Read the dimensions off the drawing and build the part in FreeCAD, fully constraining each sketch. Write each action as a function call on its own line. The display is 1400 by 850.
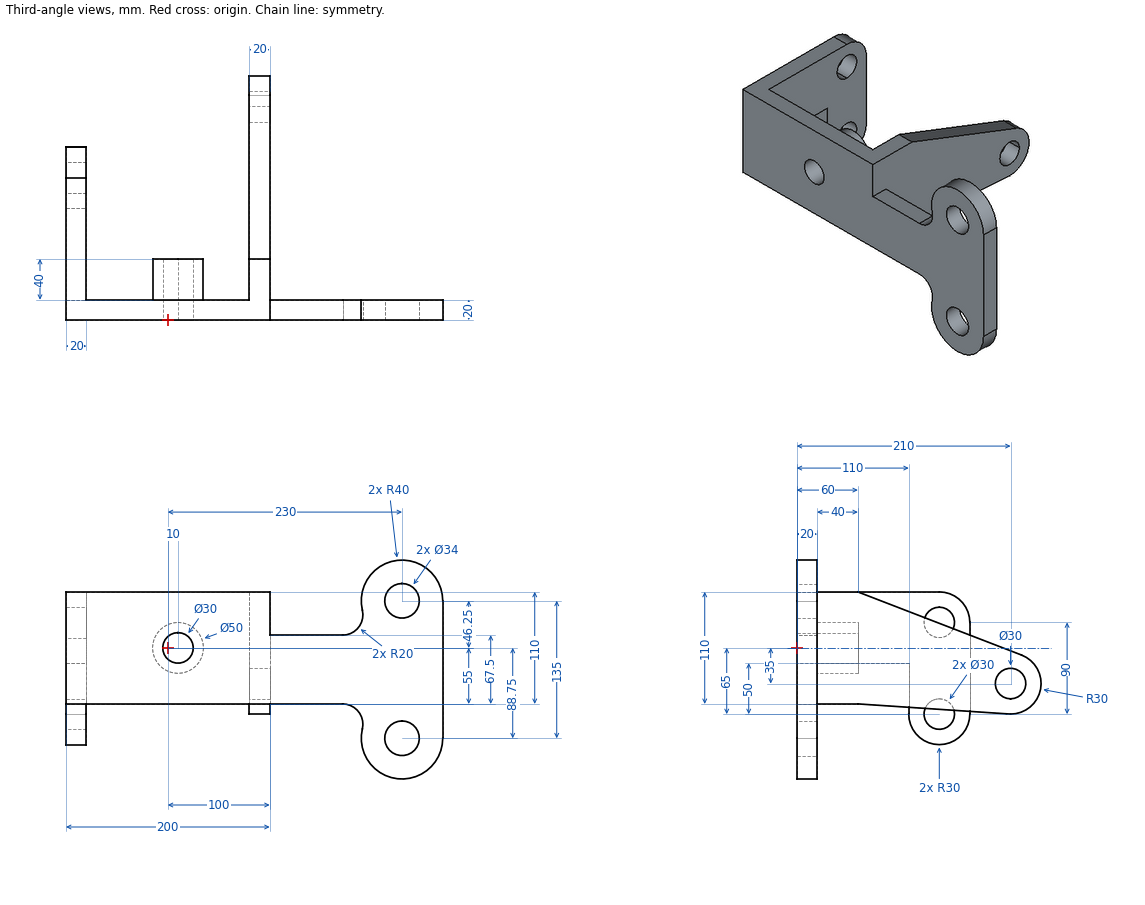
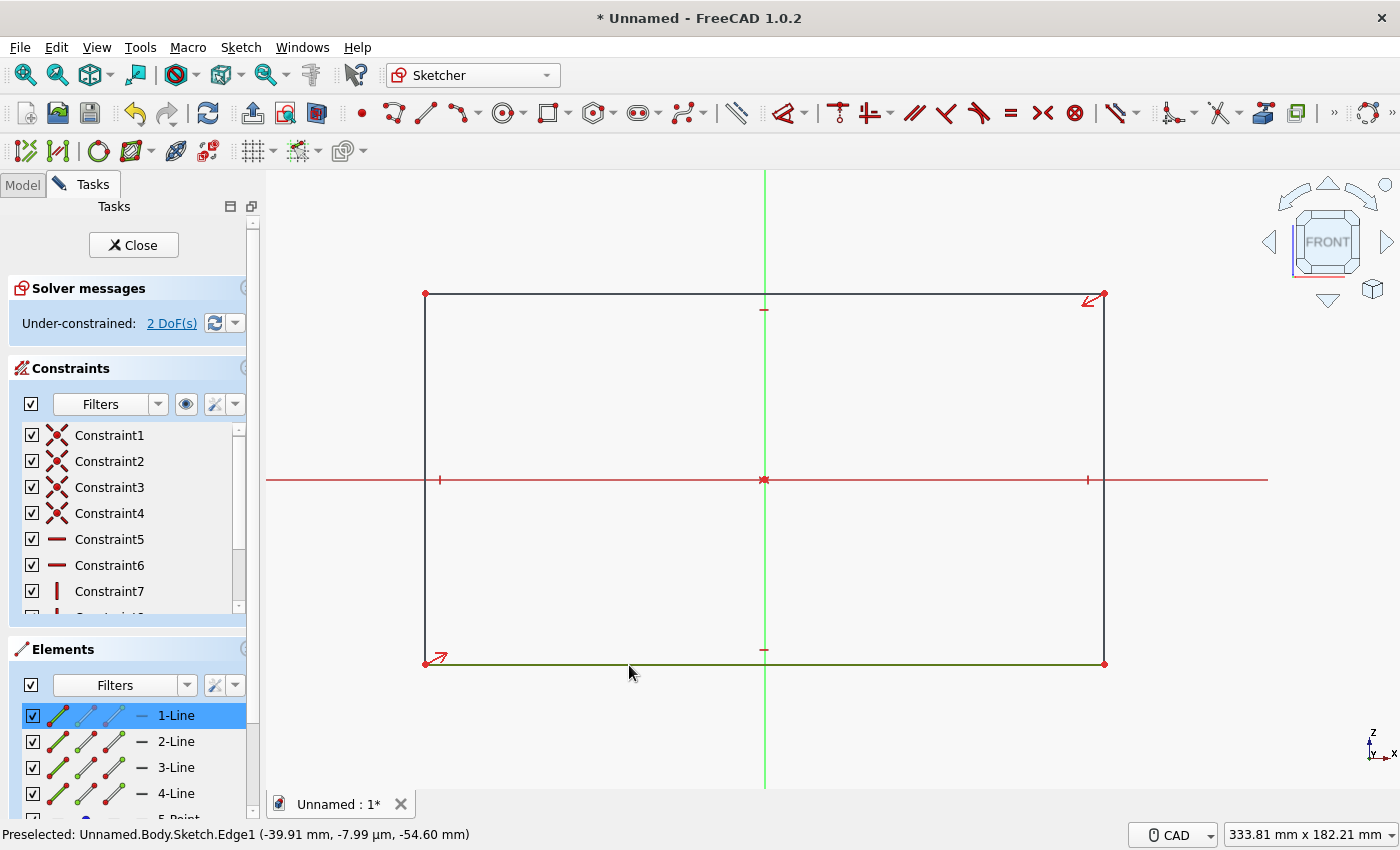
key(l)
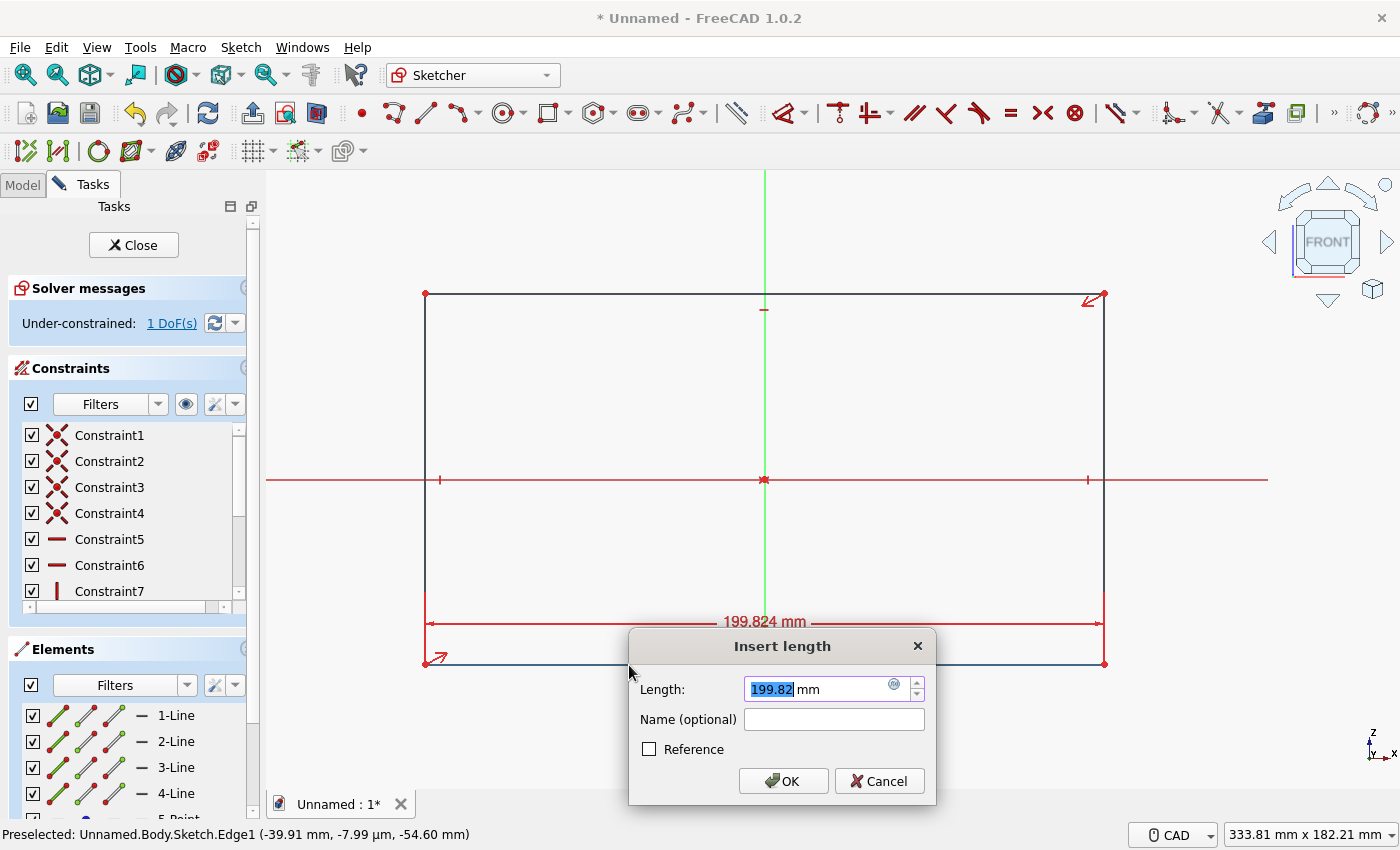
text(200)
key(Return)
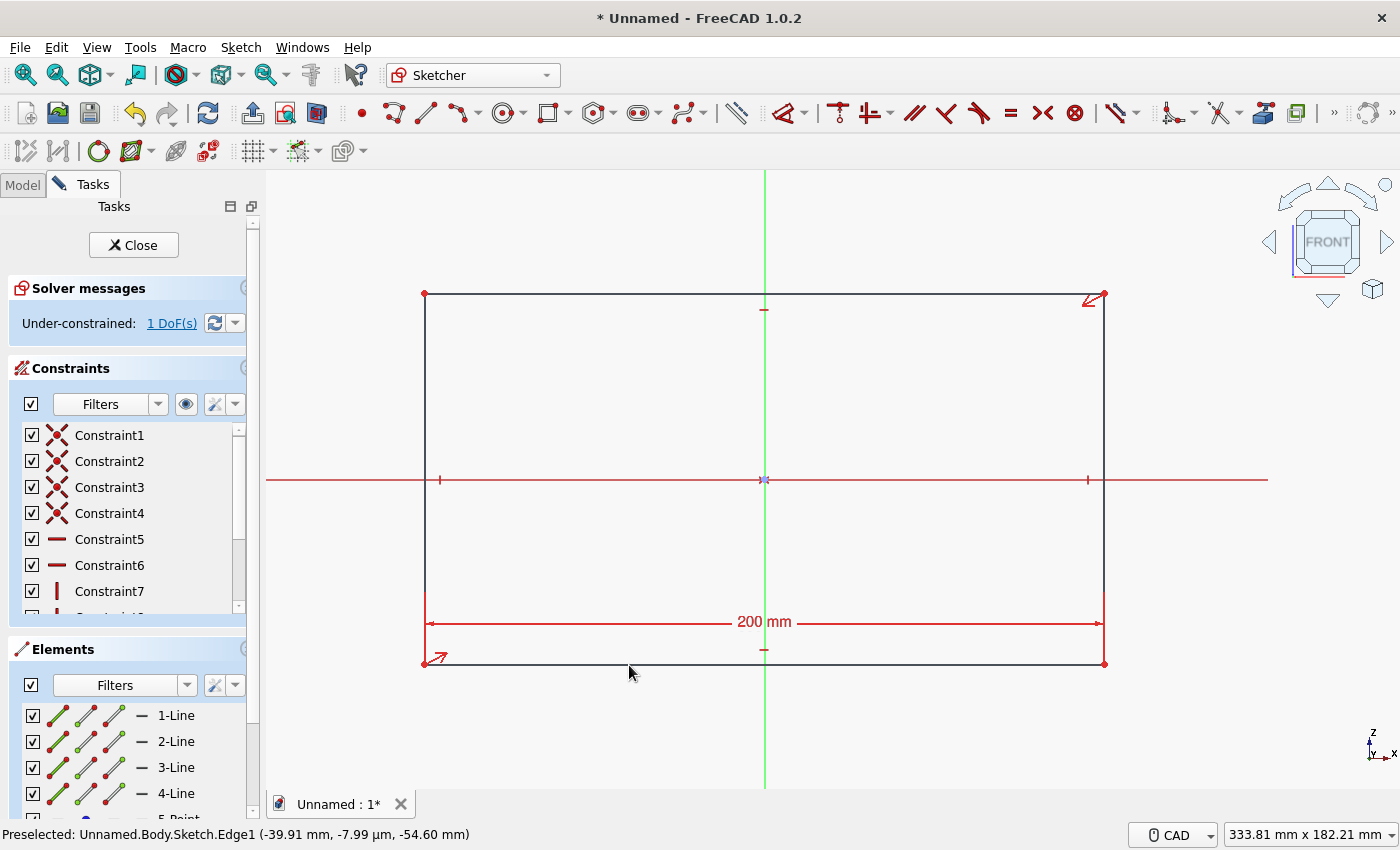
click(1104, 554)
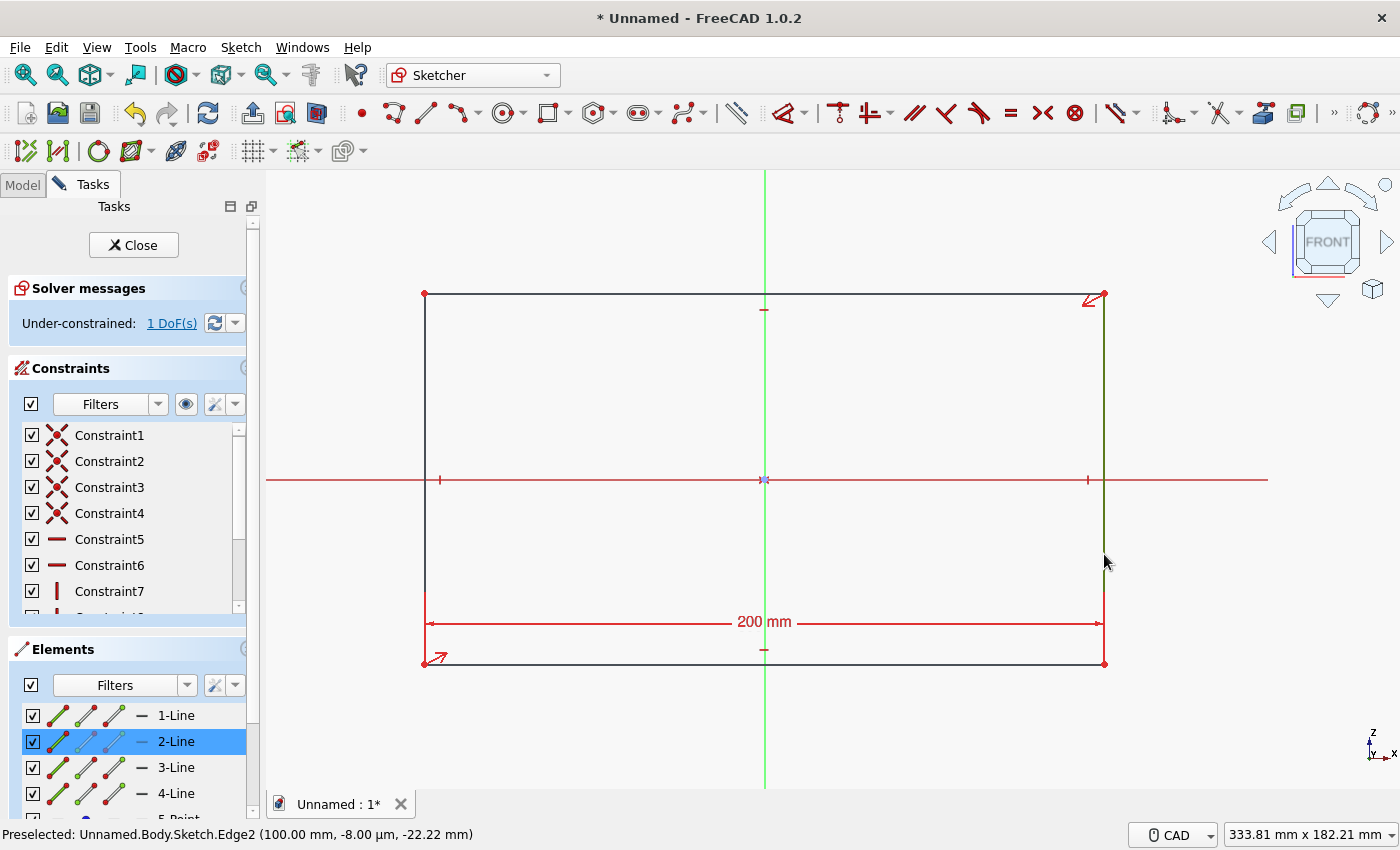
key(i)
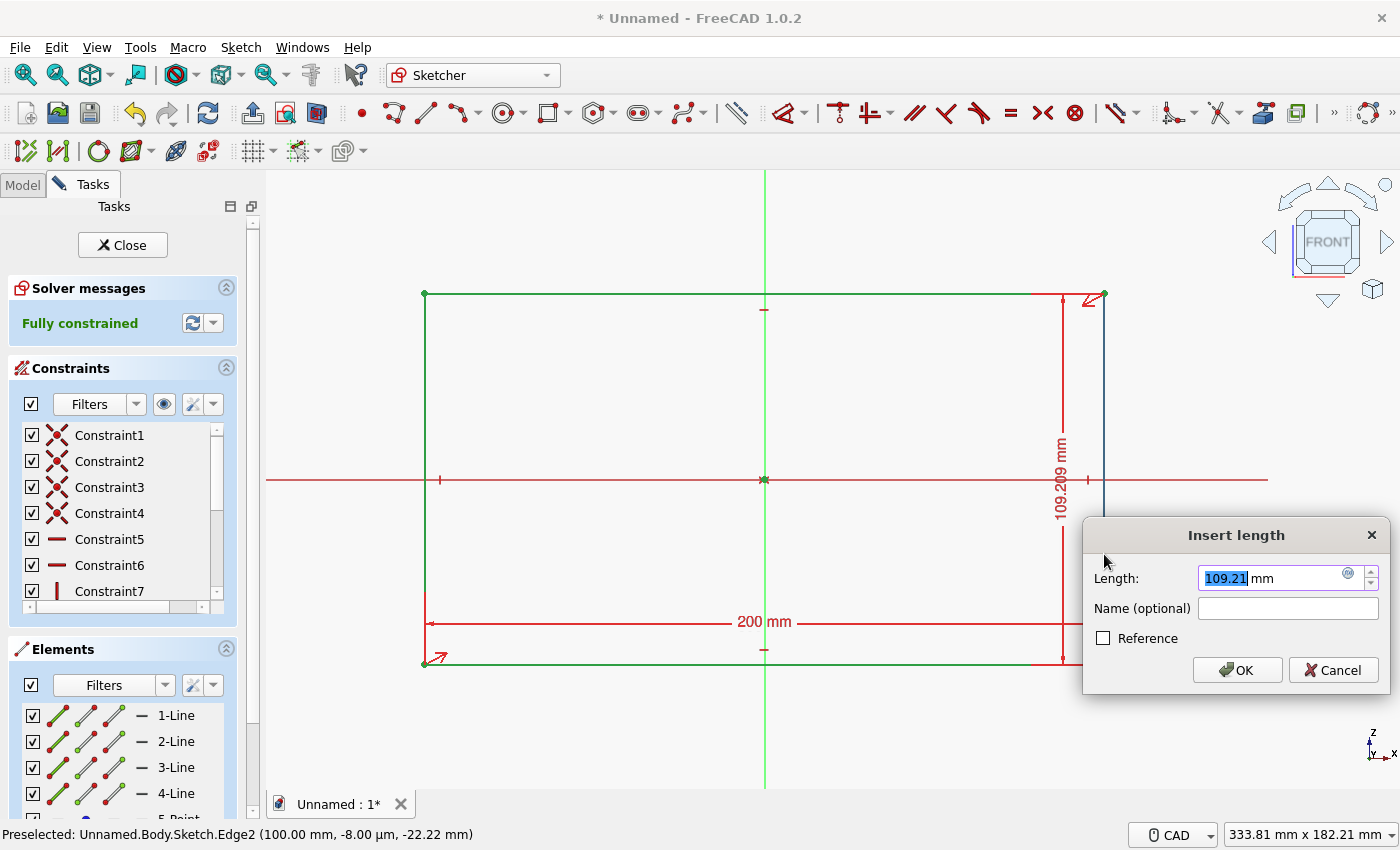
text(110)
key(Return)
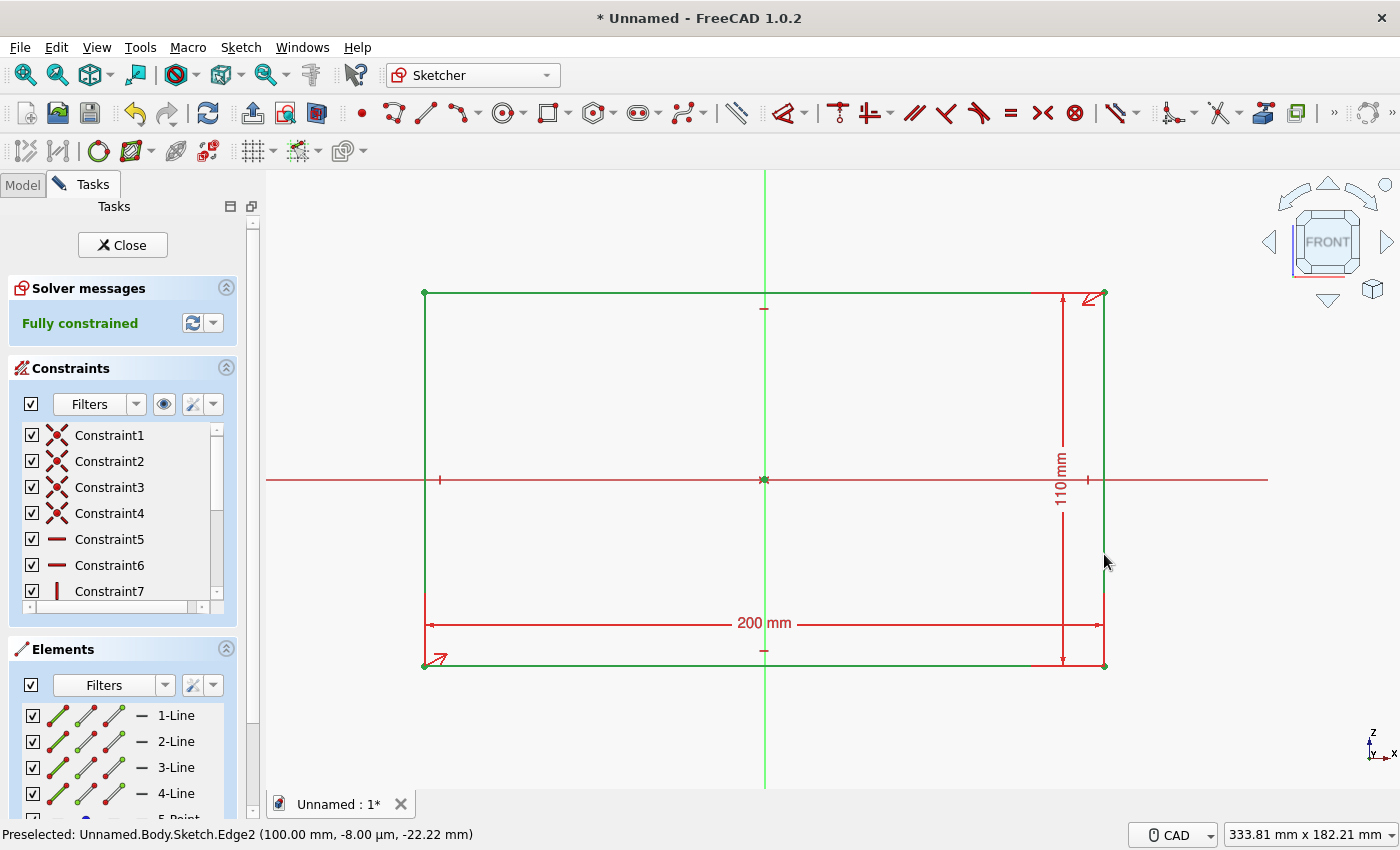
click(123, 245)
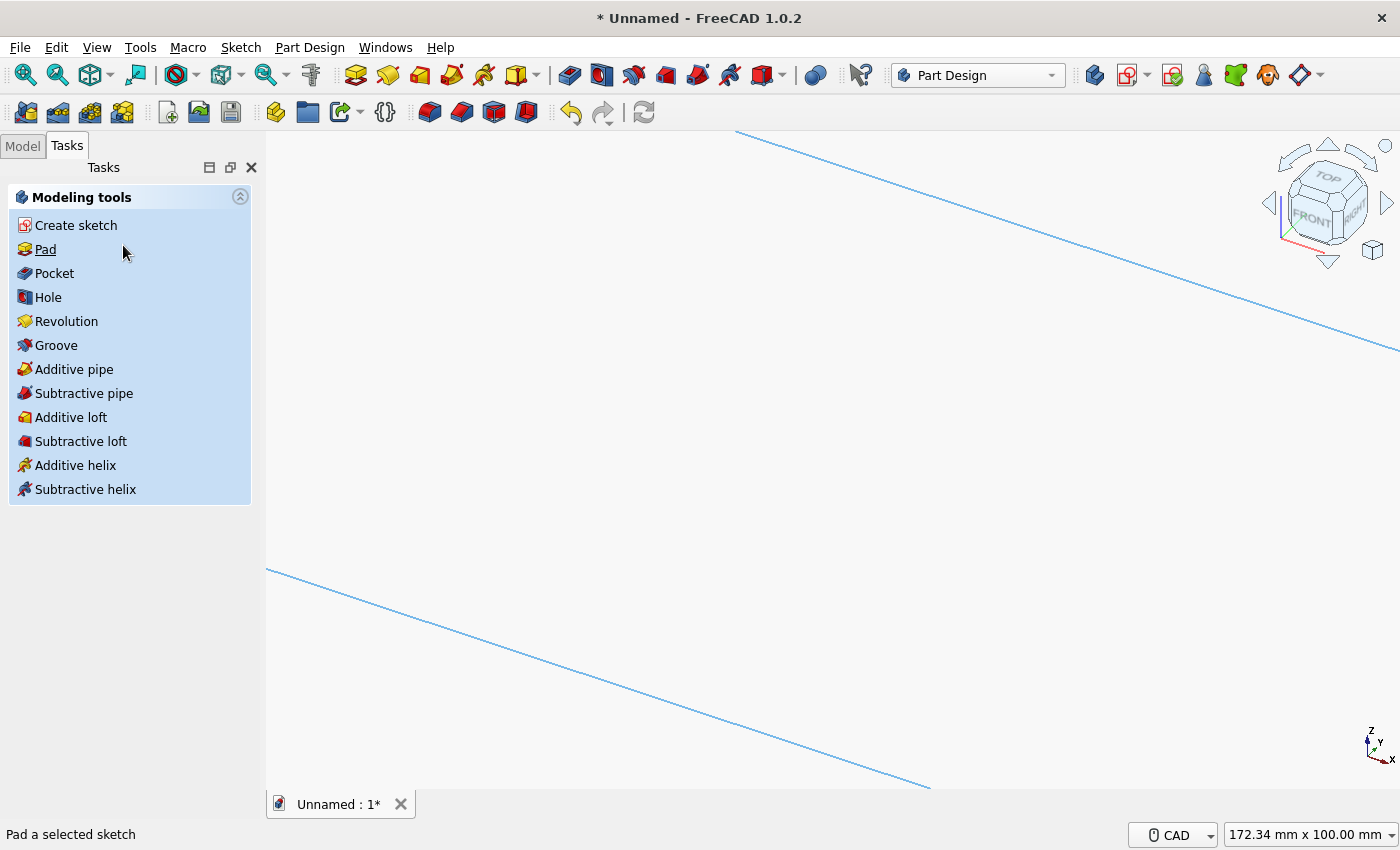
click(356, 76)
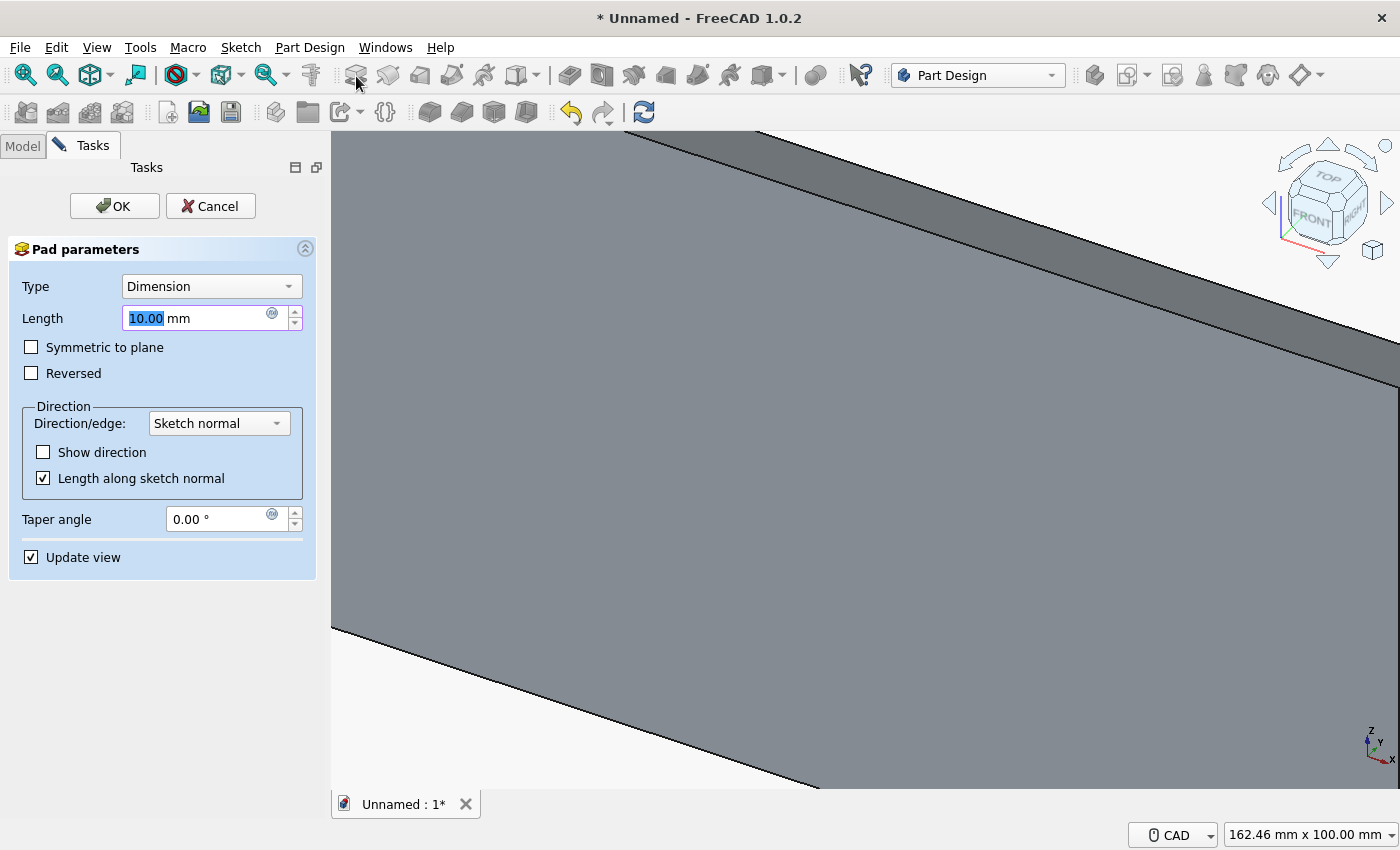
text(20)
key(Tab)